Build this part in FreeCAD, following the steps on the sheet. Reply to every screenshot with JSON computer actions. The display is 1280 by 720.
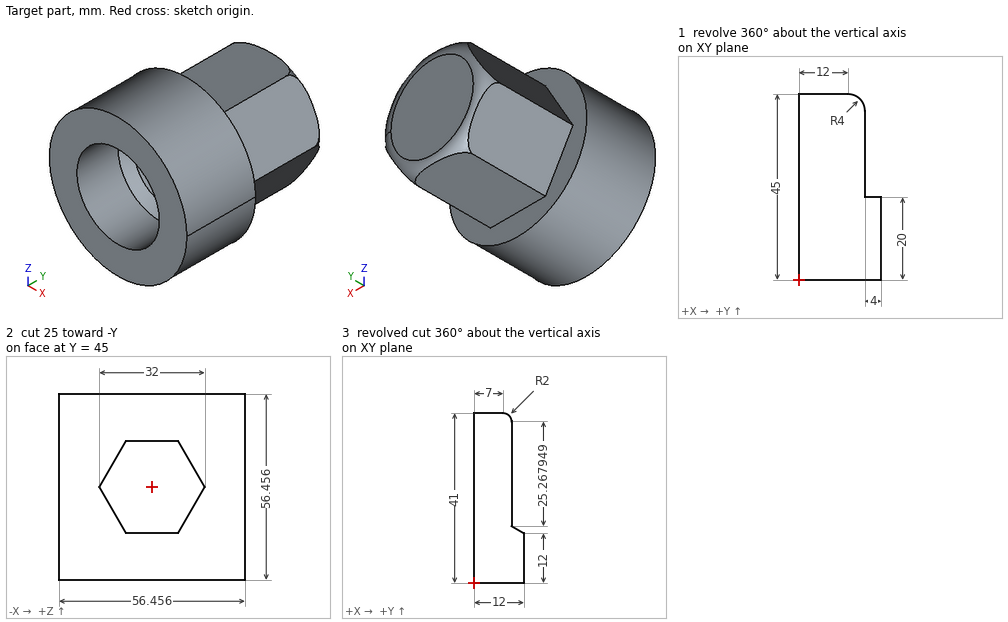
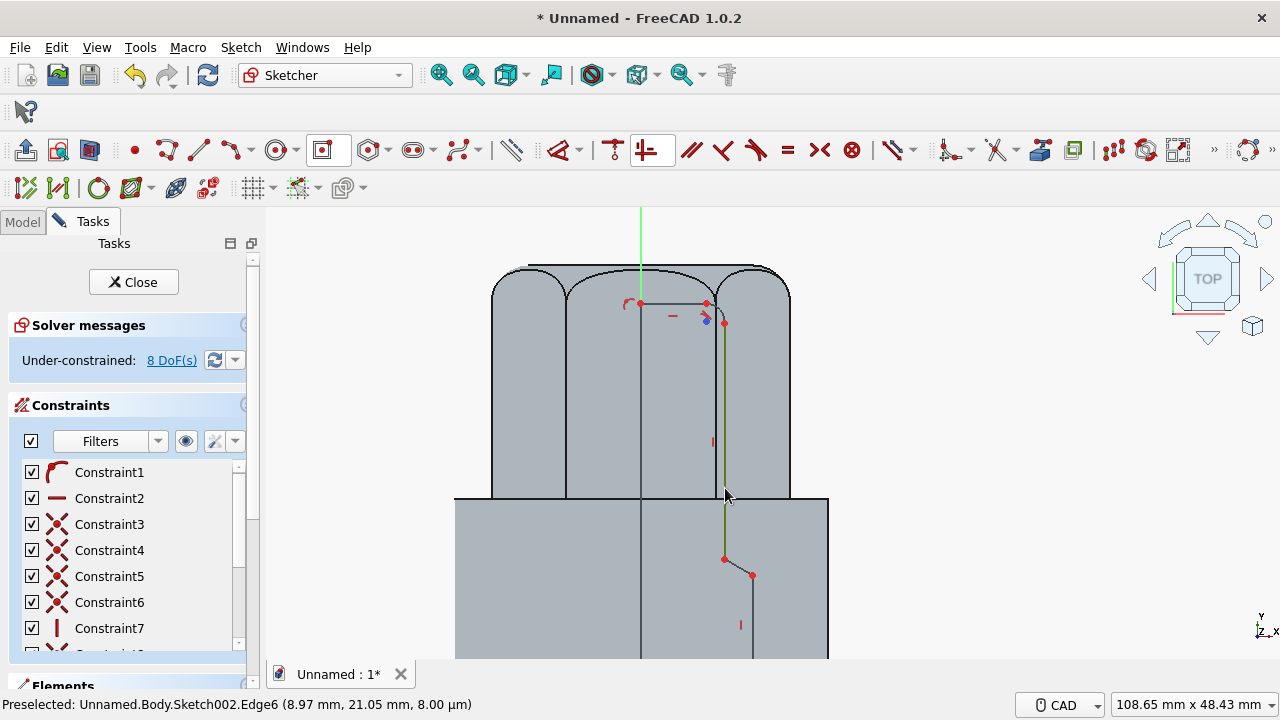
{"action": "left_click", "coordinate": [720, 310]}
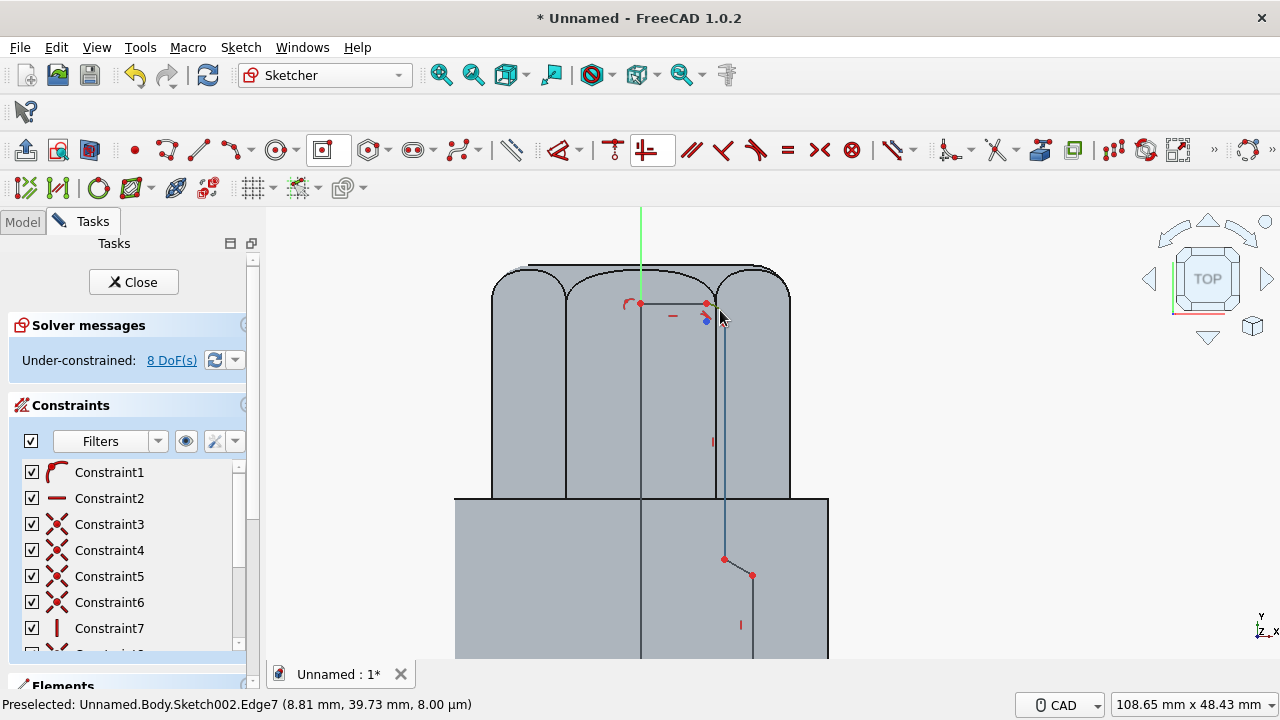
{"action": "key", "text": "t"}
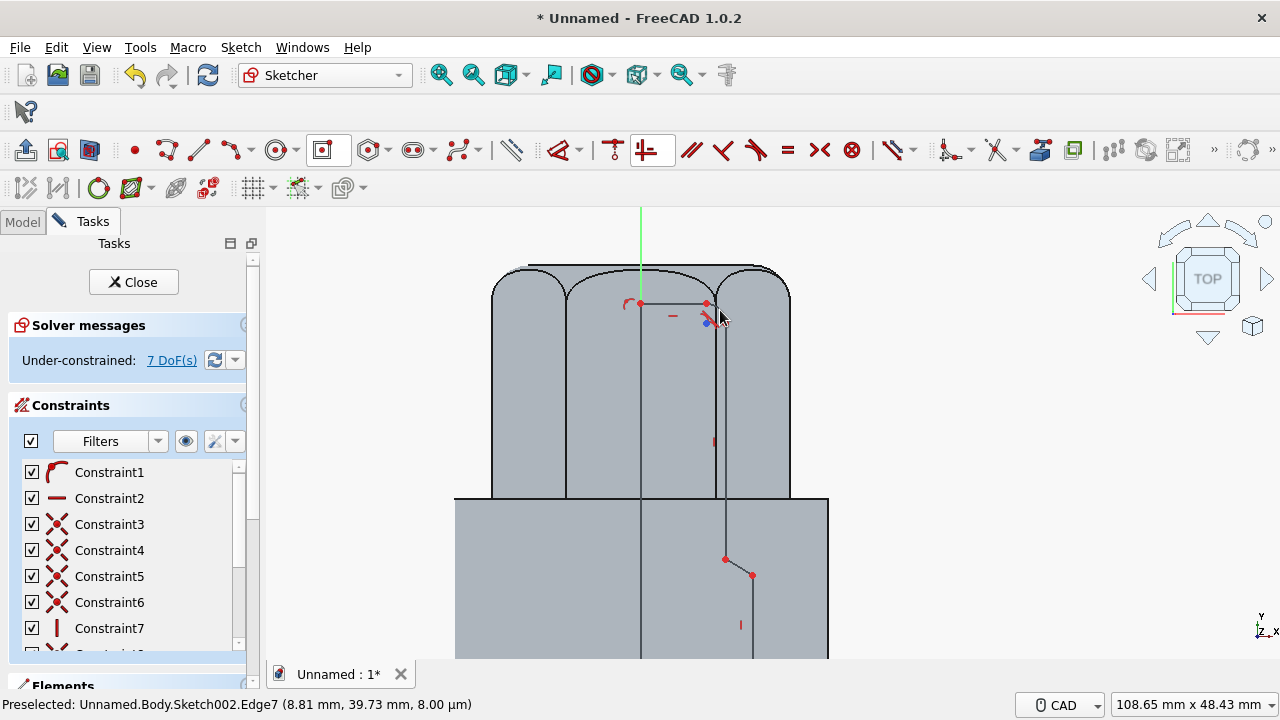
{"action": "scroll", "coordinate": [720, 309], "scroll_direction": "down", "scroll_amount": 2}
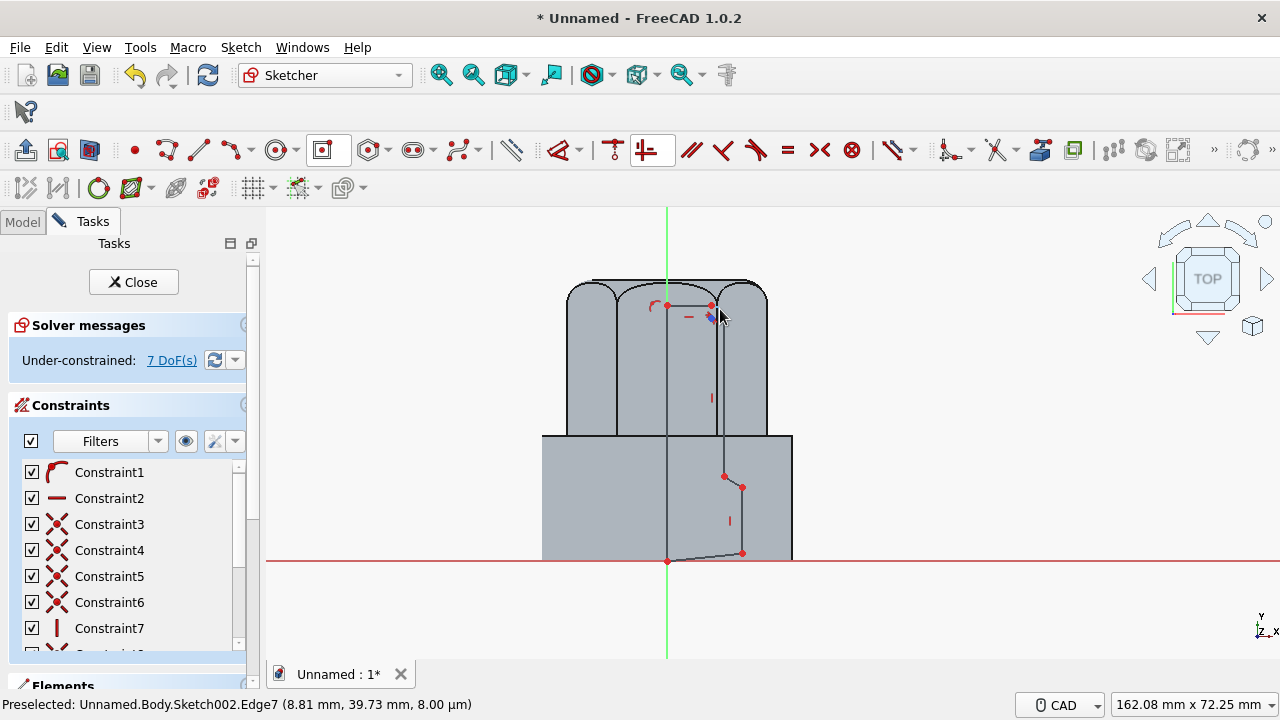
{"action": "left_click", "coordinate": [690, 559]}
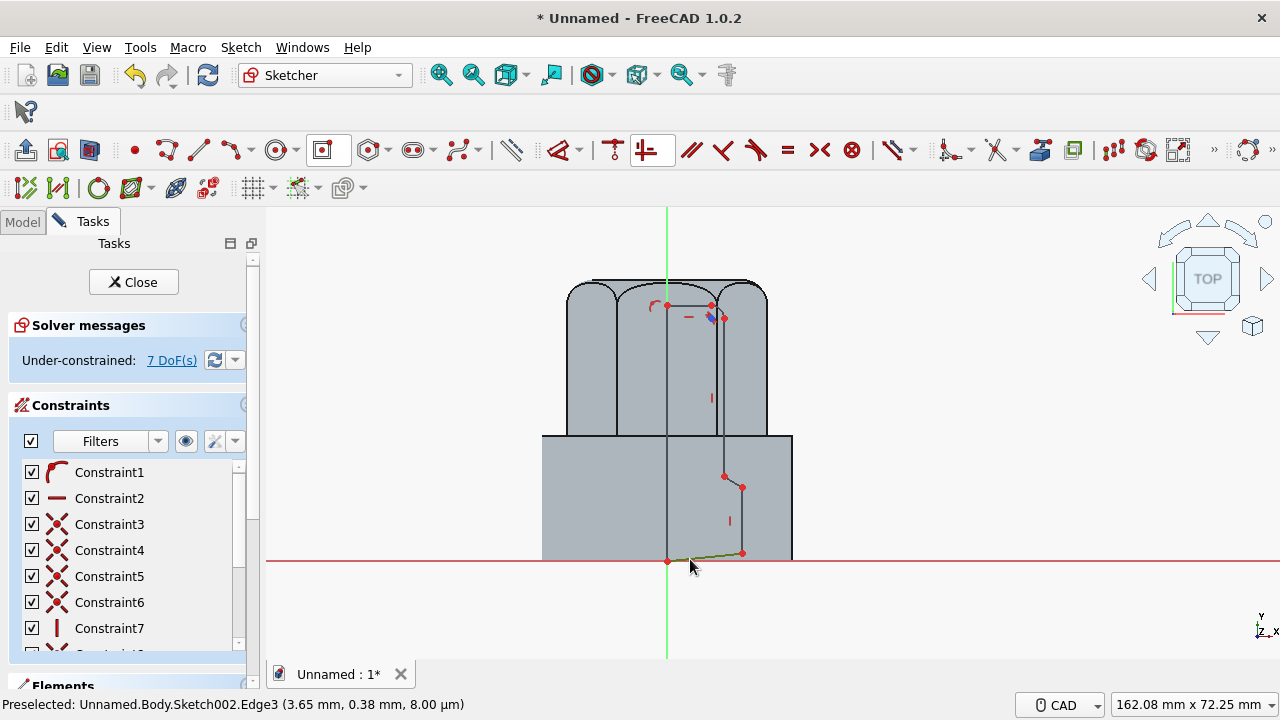
{"action": "key", "text": "h"}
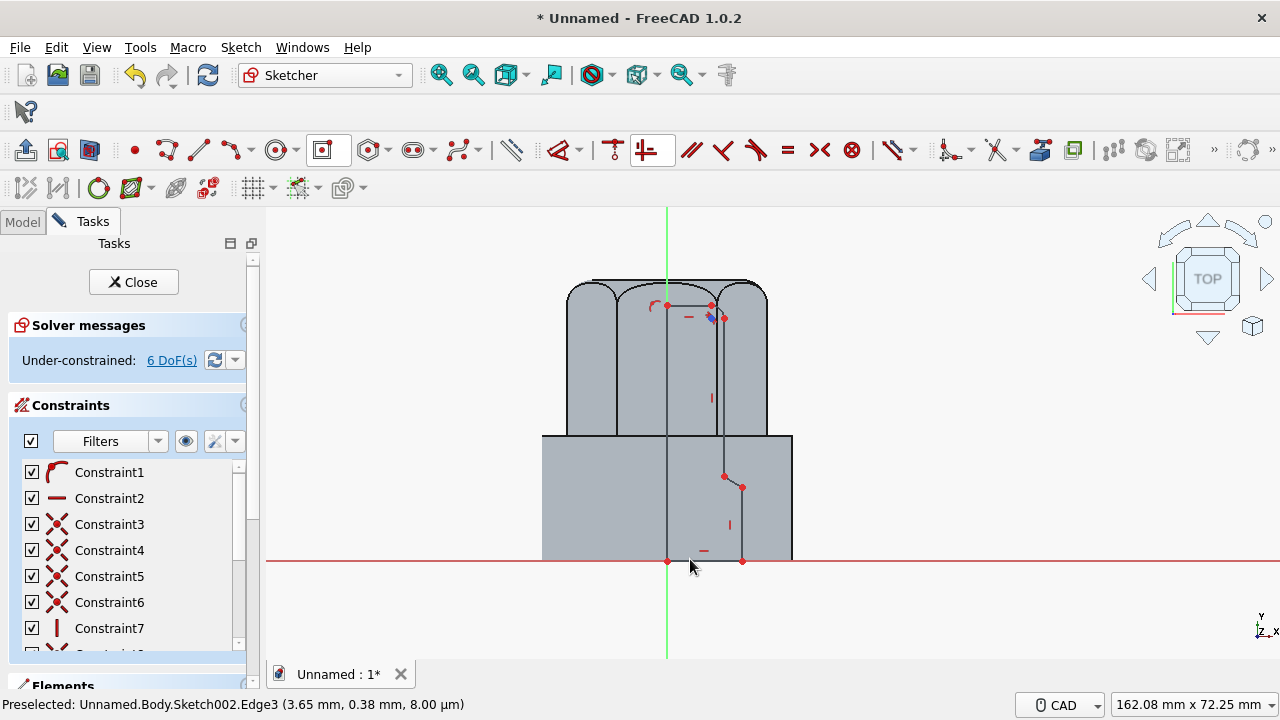
{"action": "key", "text": "d"}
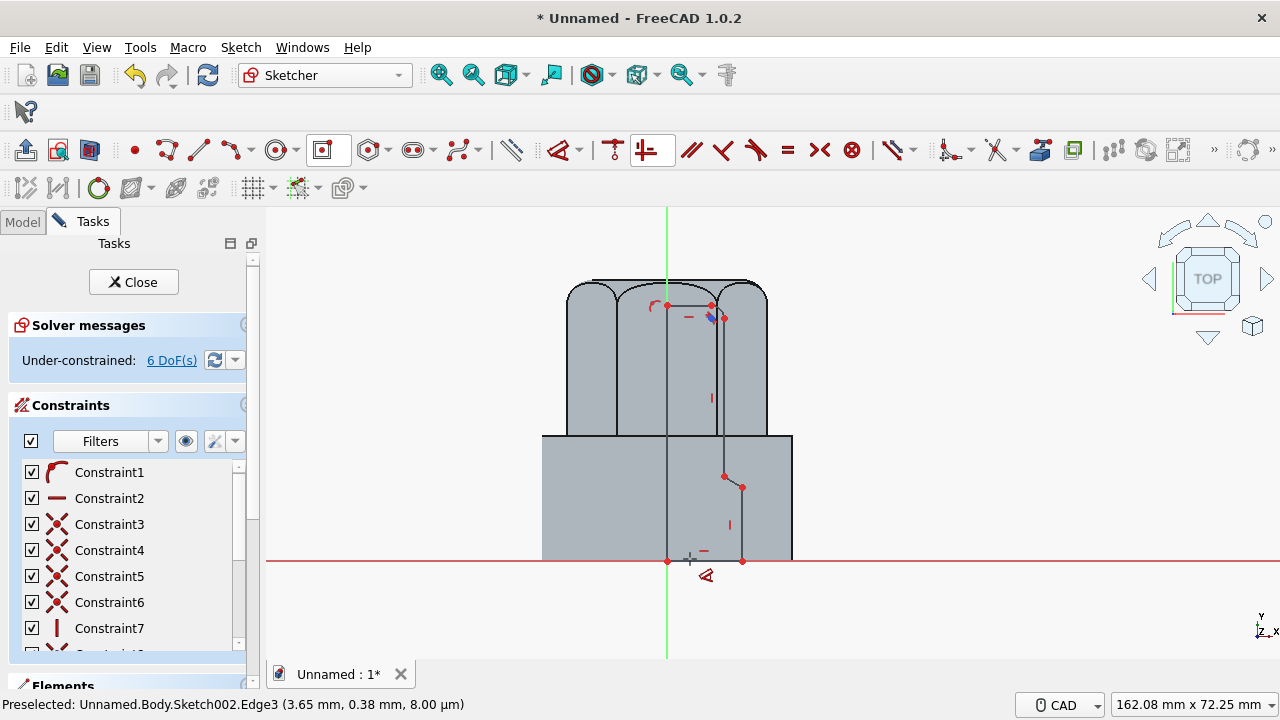
{"action": "scroll", "coordinate": [720, 309], "scroll_direction": "up", "scroll_amount": 6}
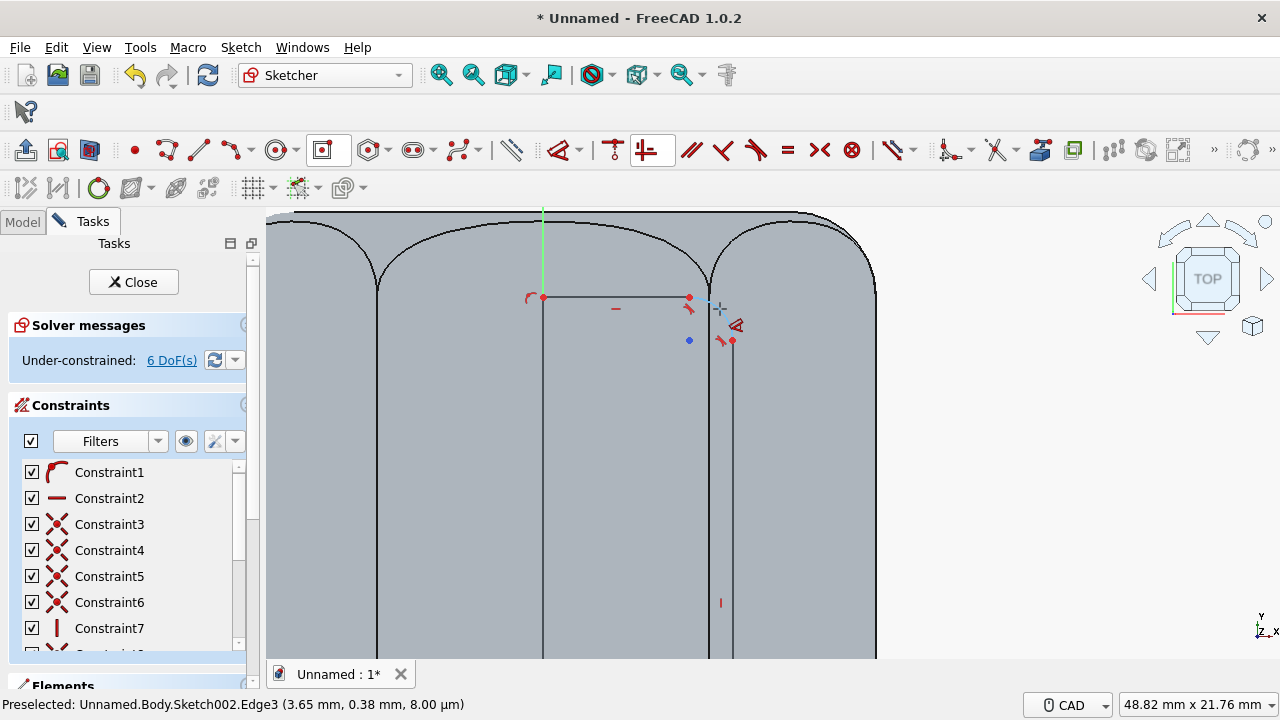
{"action": "left_click", "coordinate": [720, 310]}
{"action": "left_click", "coordinate": [743, 287]}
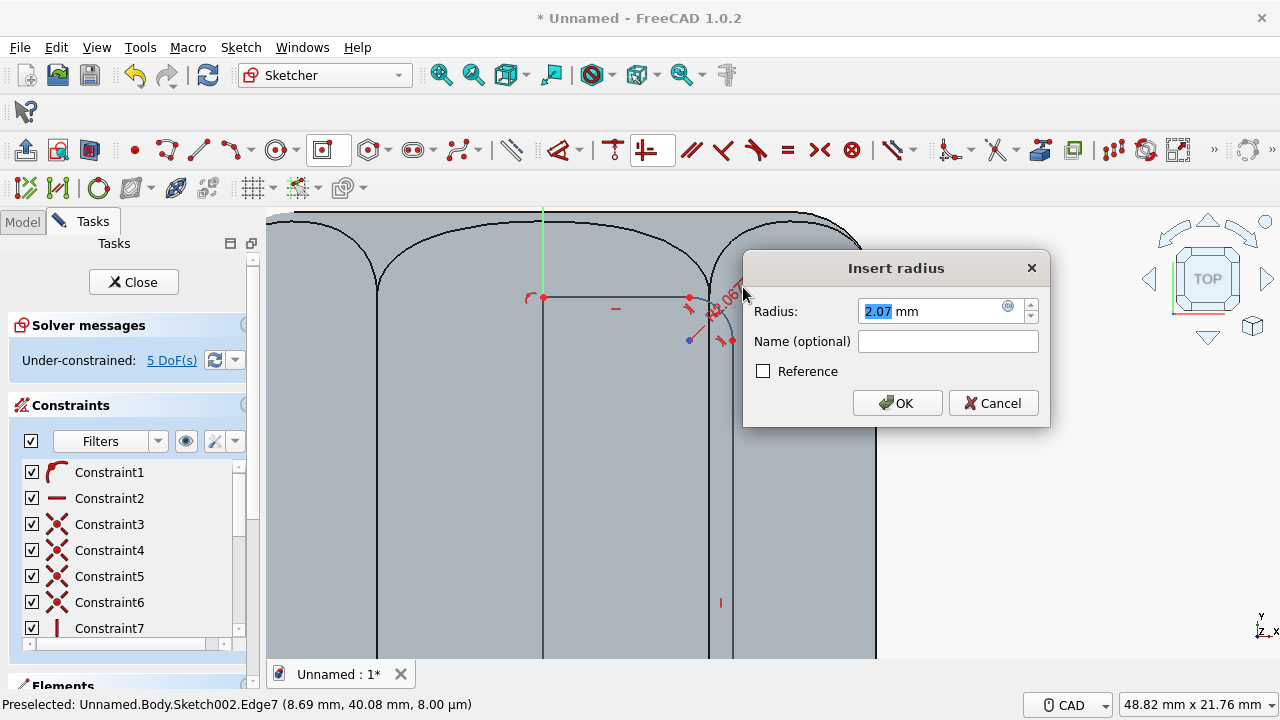
{"action": "type", "text": "2"}
{"action": "key", "text": "Return"}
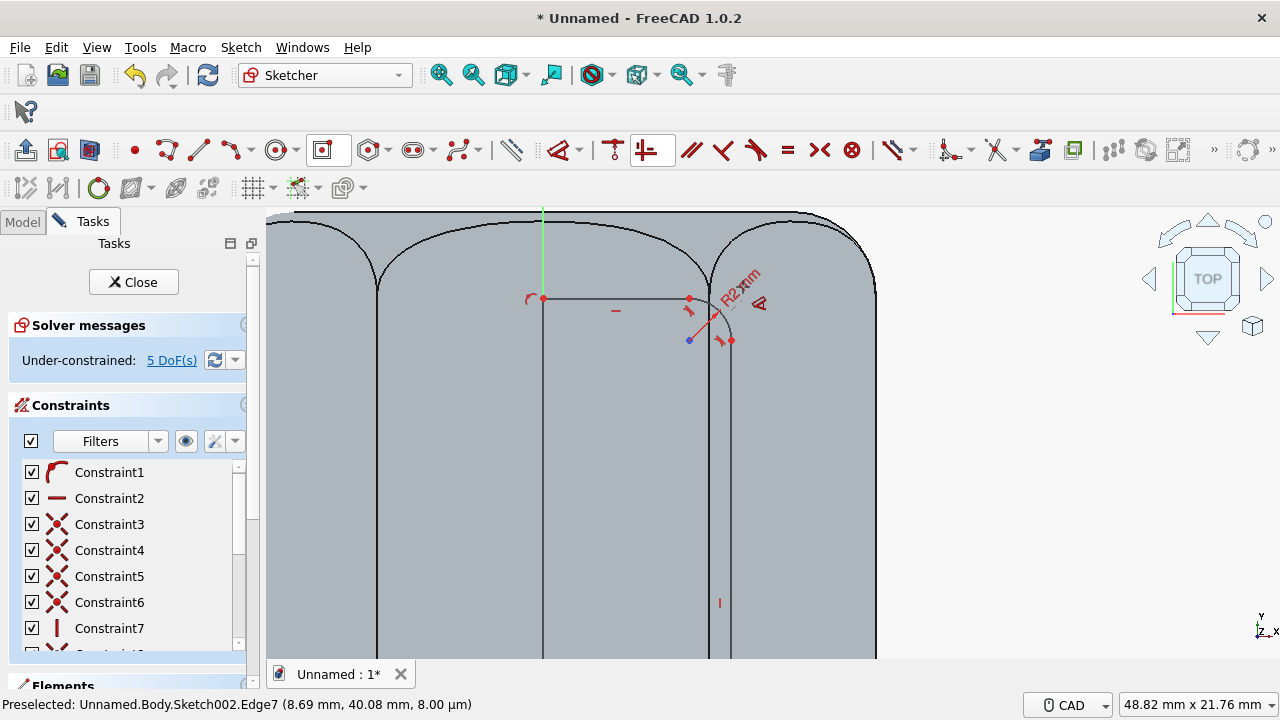
{"action": "left_click", "coordinate": [646, 299]}
{"action": "left_click", "coordinate": [617, 265]}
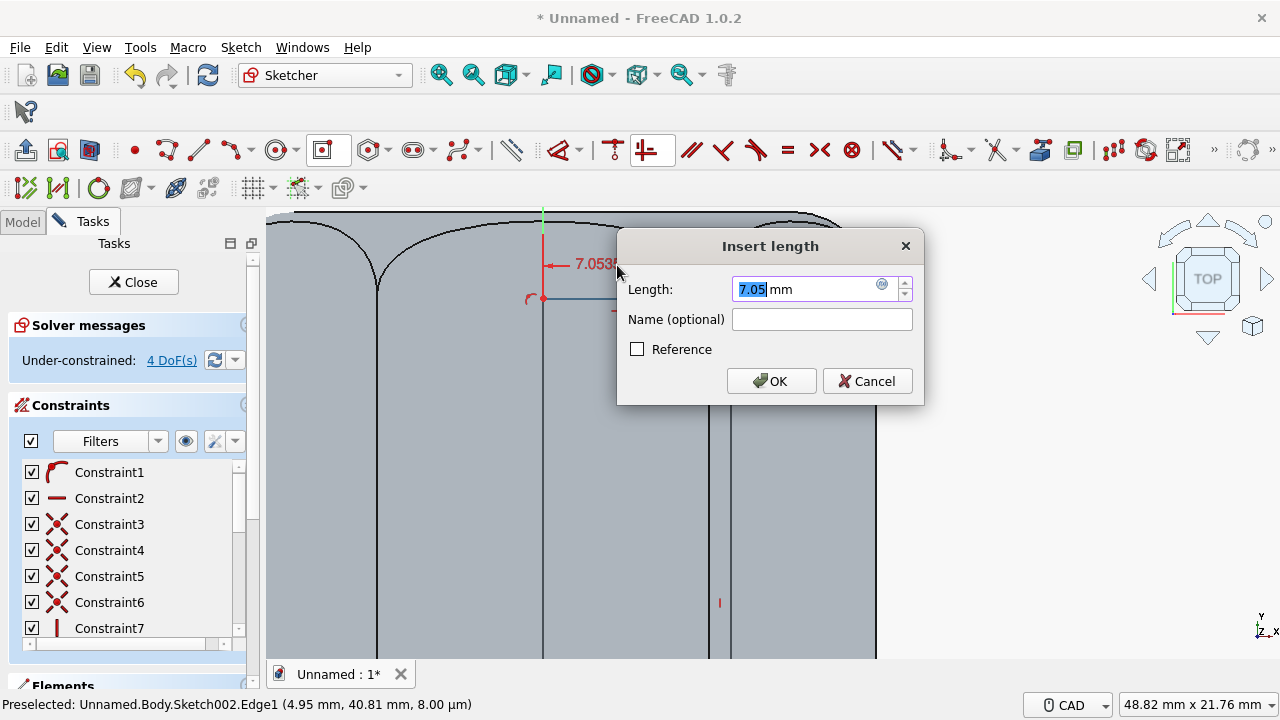
{"action": "type", "text": "7"}
{"action": "key", "text": "Return"}